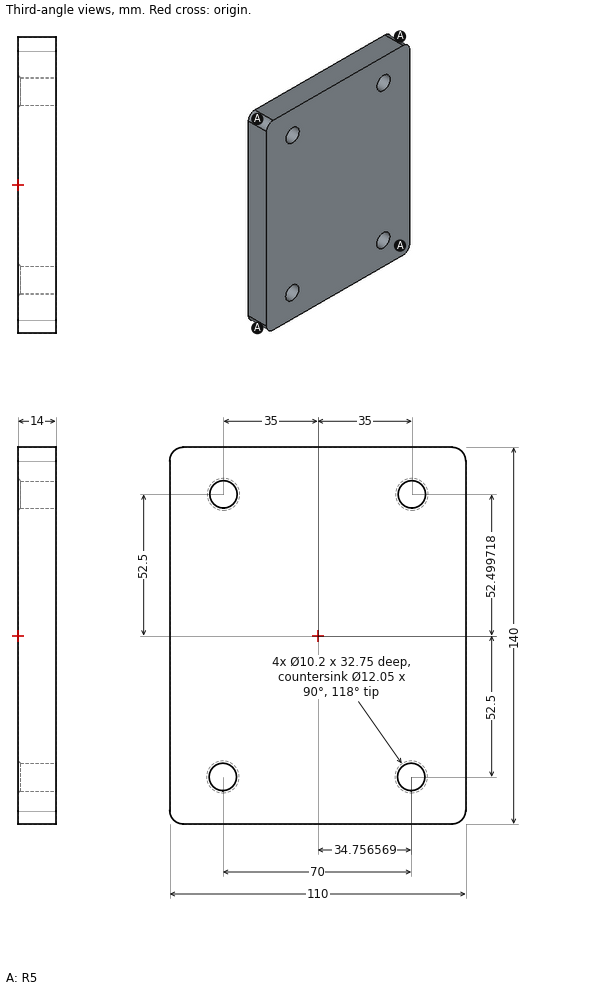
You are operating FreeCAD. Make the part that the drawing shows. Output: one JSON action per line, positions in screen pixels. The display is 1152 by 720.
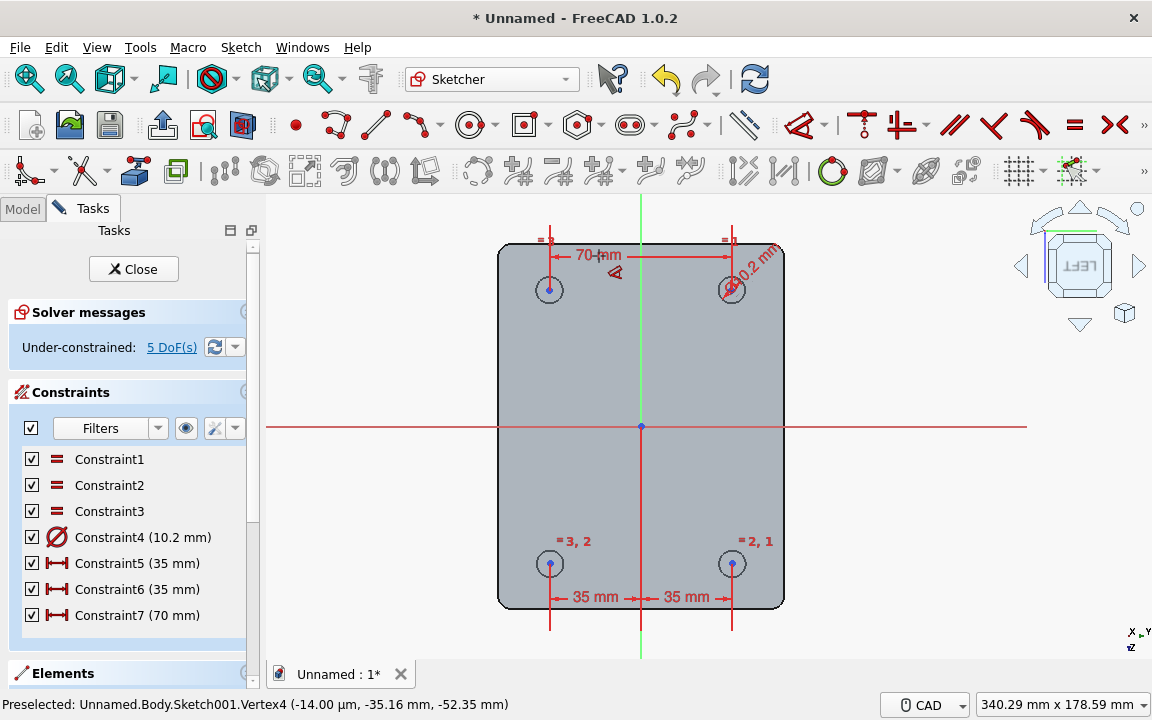
{"action": "left_click", "coordinate": [732, 290]}
{"action": "left_click", "coordinate": [766, 358]}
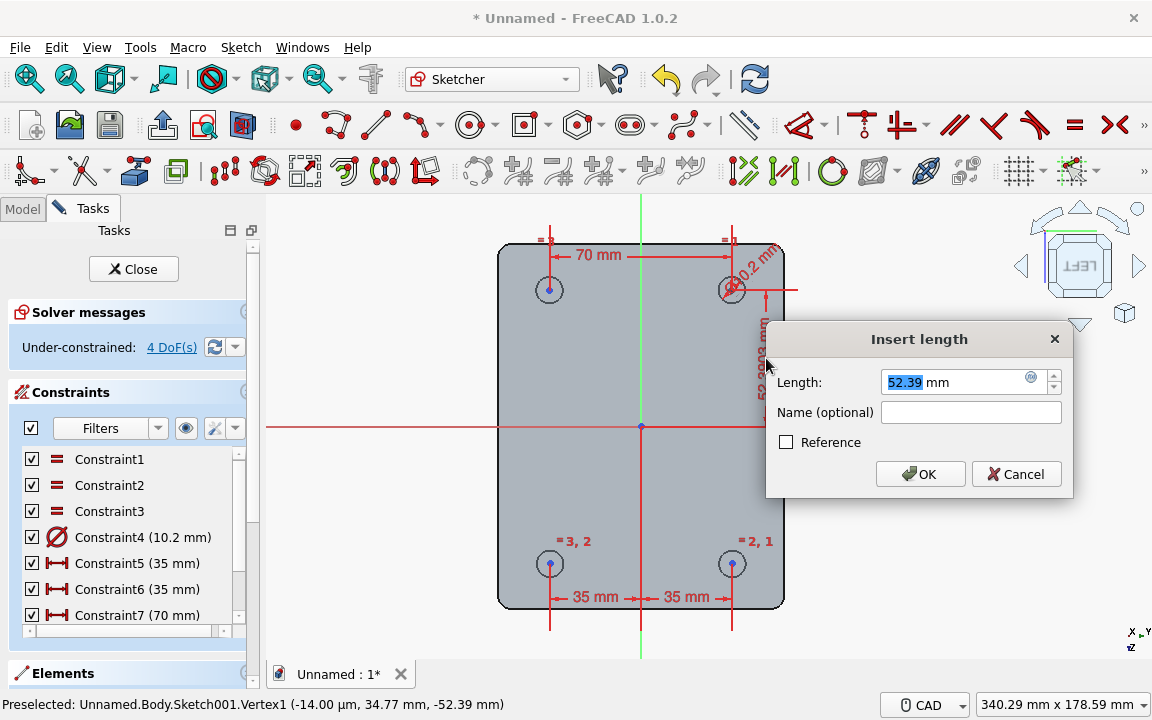
{"action": "type", "text": "52.5"}
{"action": "key", "text": "Return"}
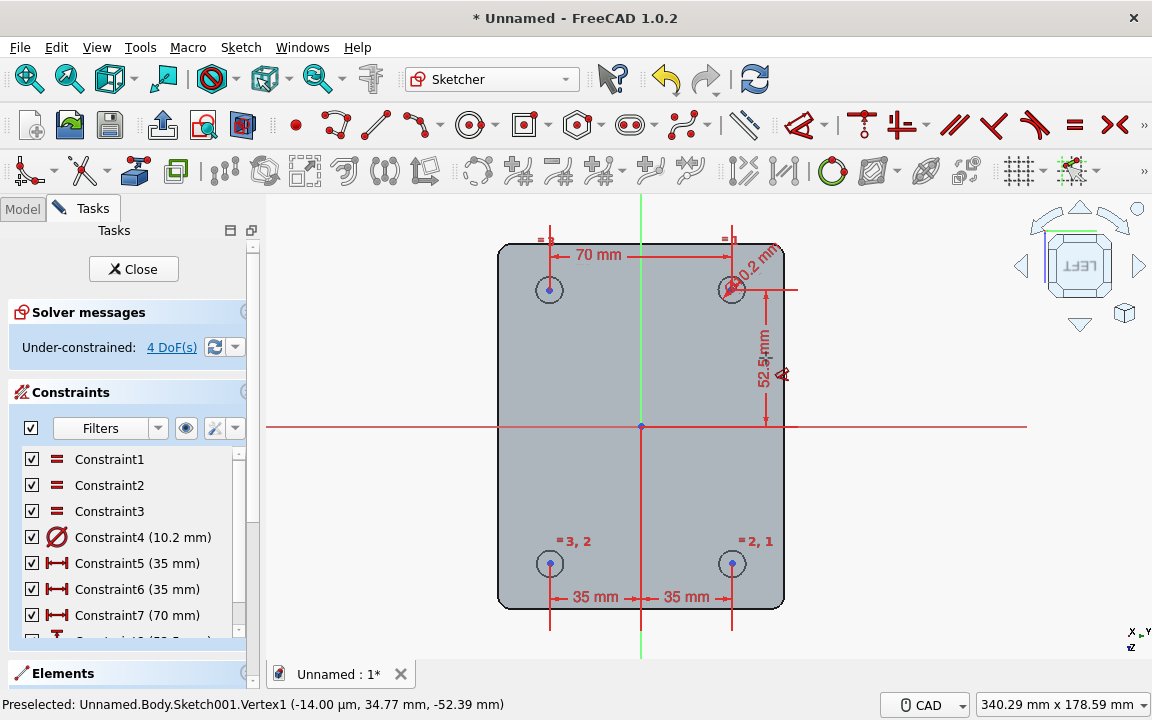
{"action": "left_click", "coordinate": [550, 564]}
{"action": "left_click", "coordinate": [516, 495]}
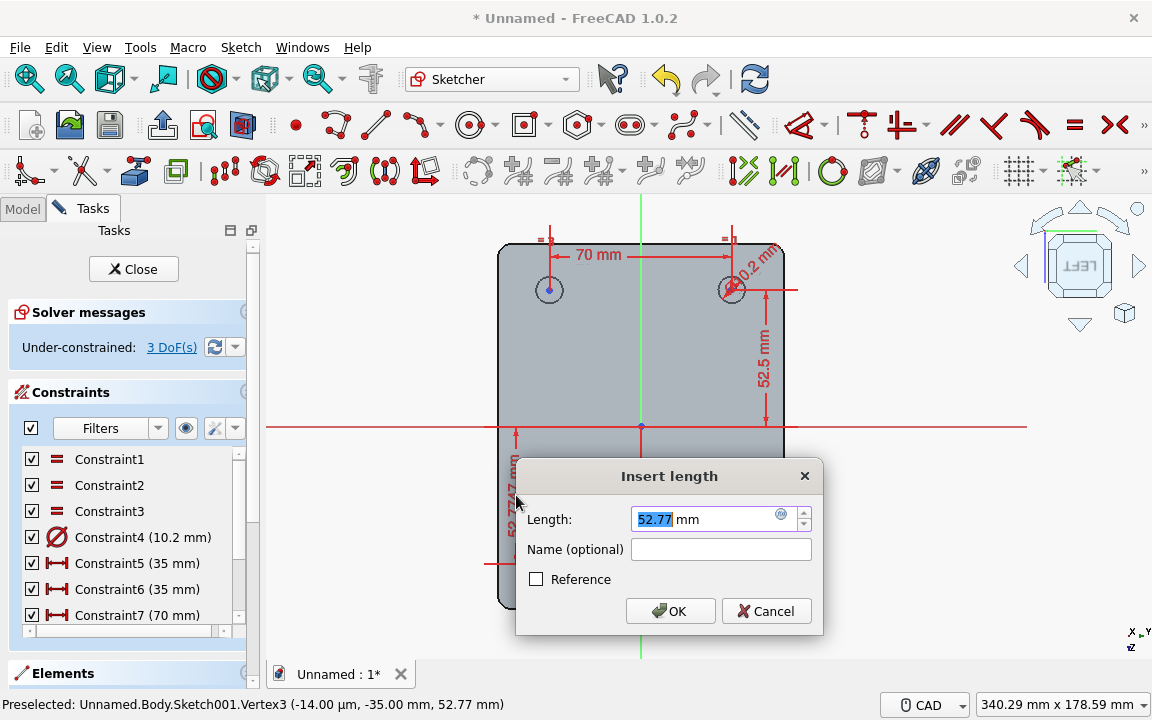
{"action": "type", "text": "52.5"}
{"action": "key", "text": "Return"}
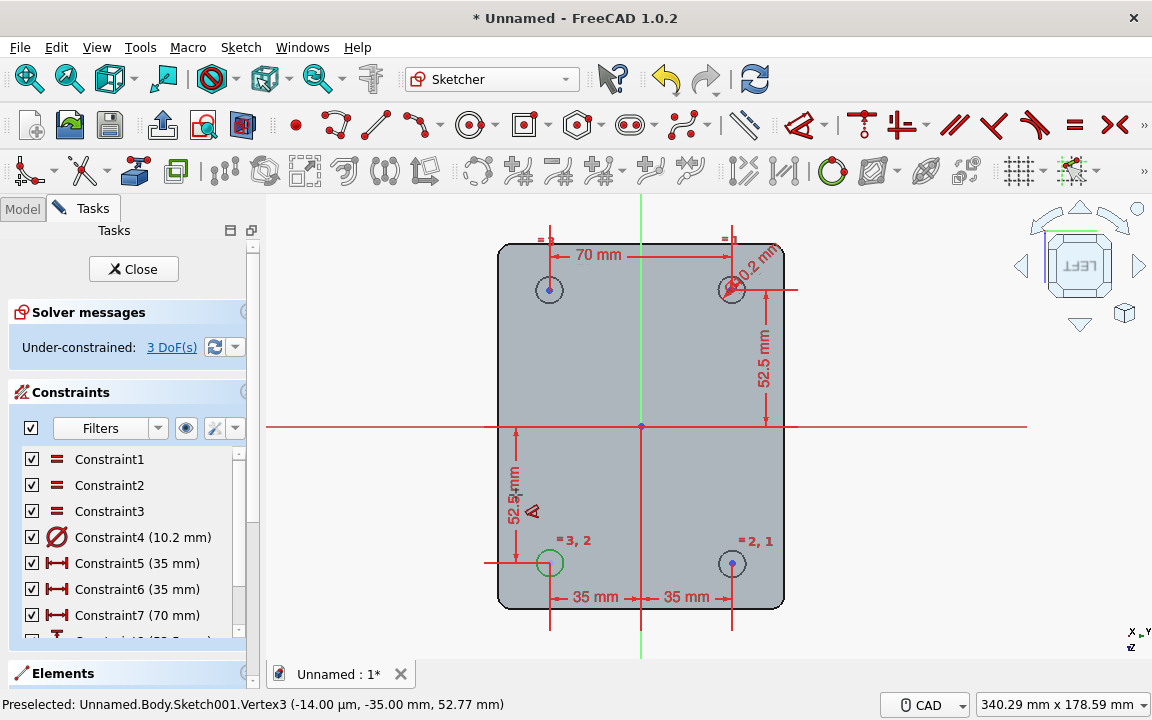
{"action": "left_click", "coordinate": [550, 290]}
{"action": "left_click", "coordinate": [516, 358]}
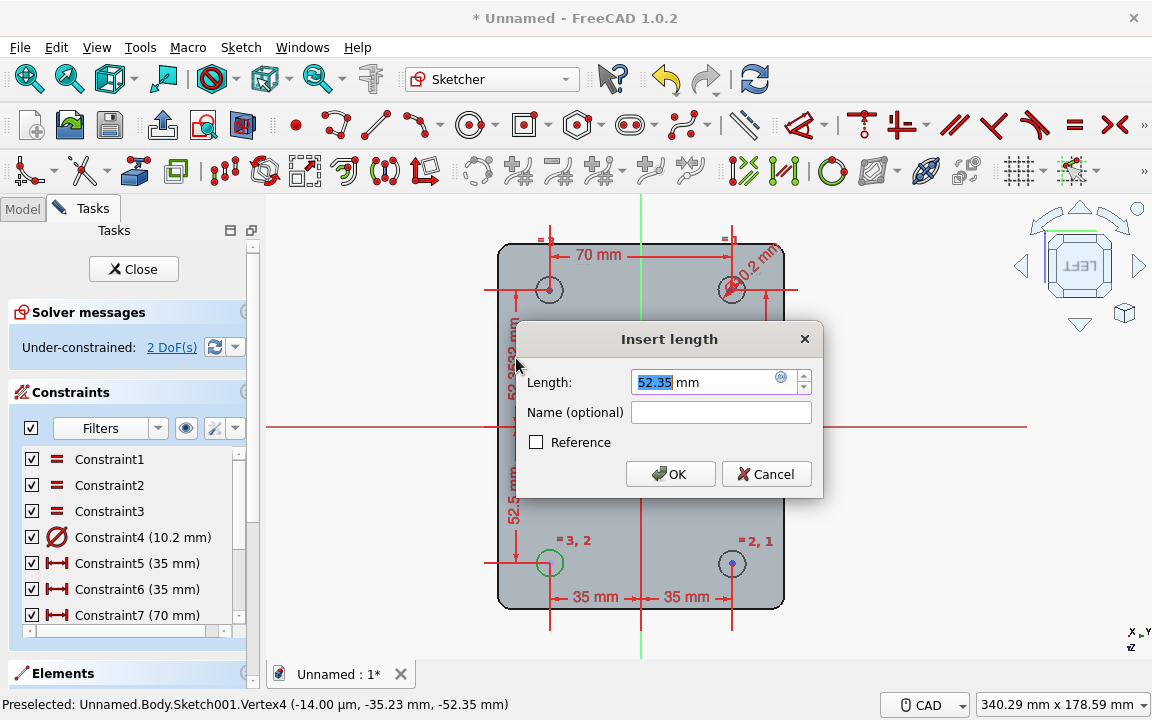
{"action": "type", "text": "52.5"}
{"action": "key", "text": "Return"}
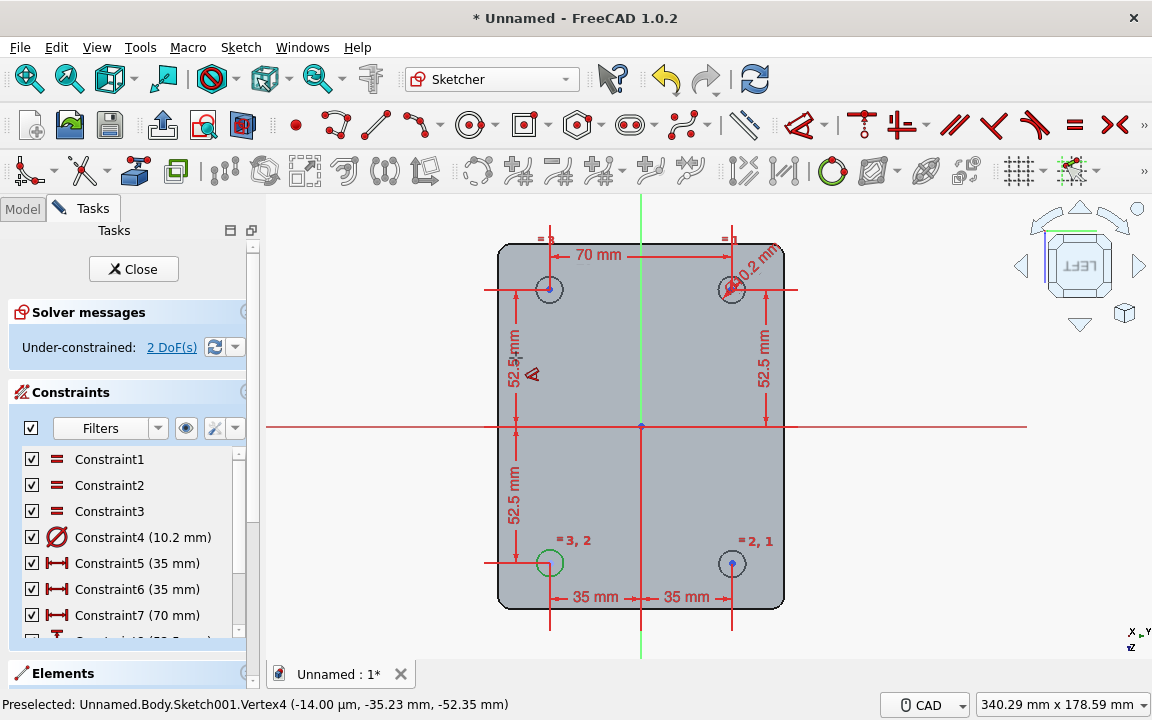
{"action": "left_click", "coordinate": [732, 290]}
{"action": "left_click", "coordinate": [687, 460]}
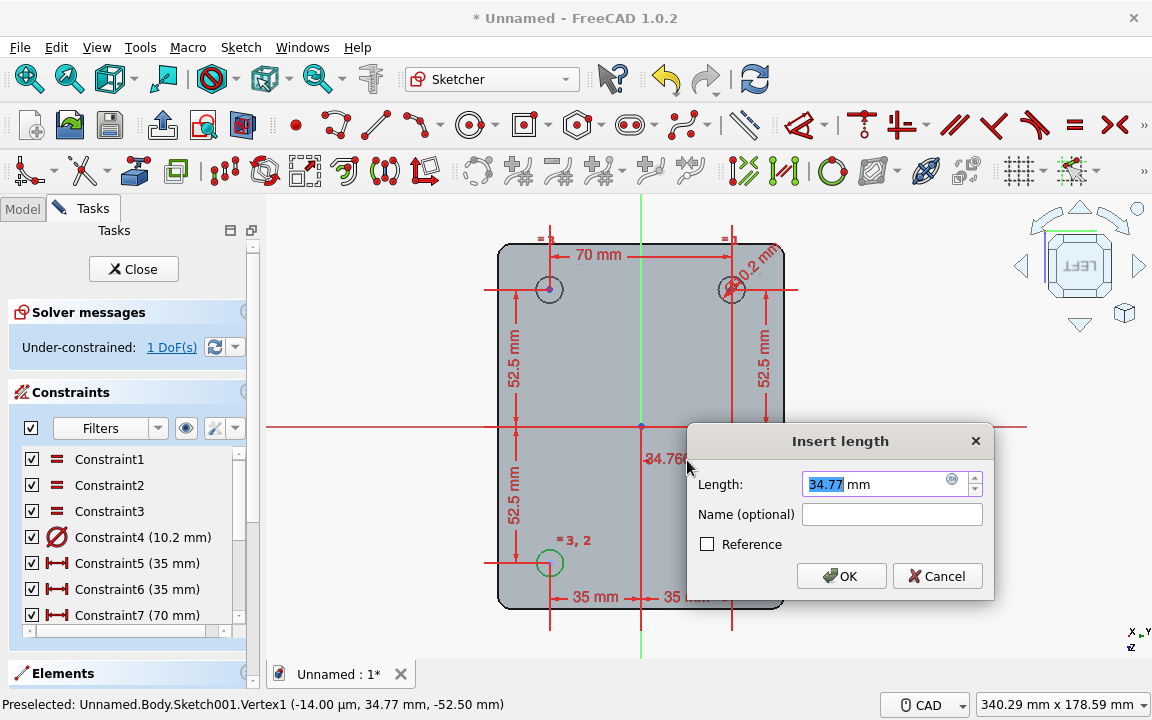
{"action": "type", "text": "34.756569"}
{"action": "key", "text": "Return"}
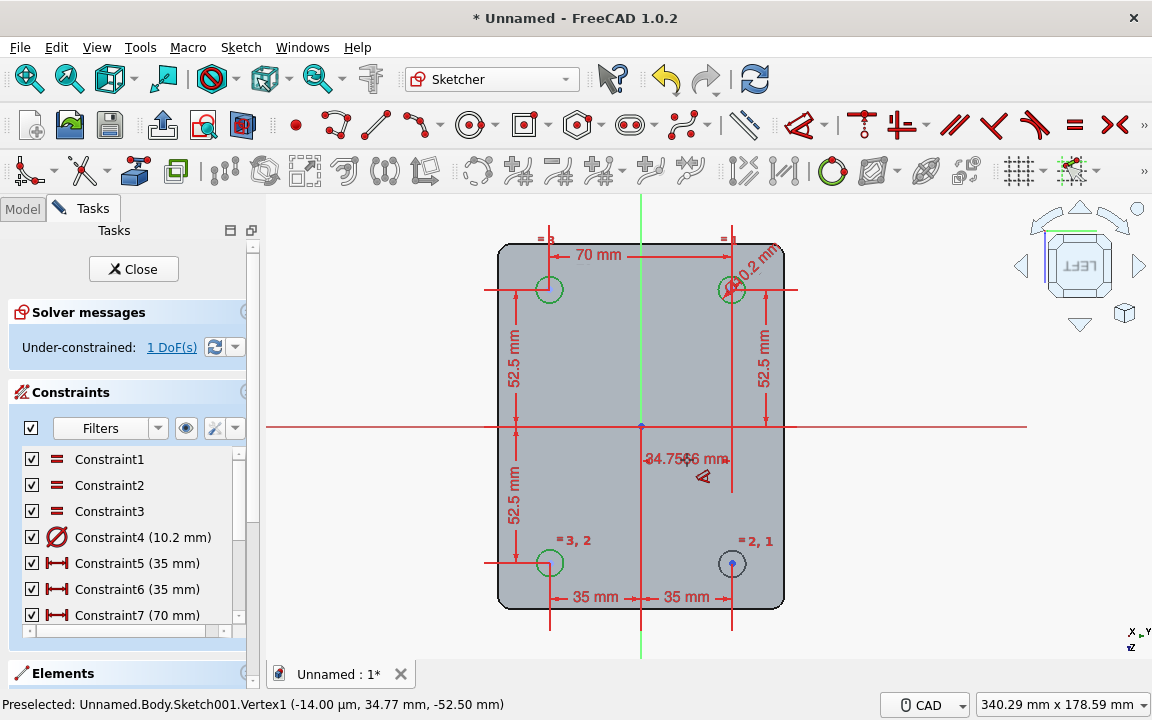
{"action": "left_click", "coordinate": [732, 564]}
{"action": "left_click", "coordinate": [766, 495]}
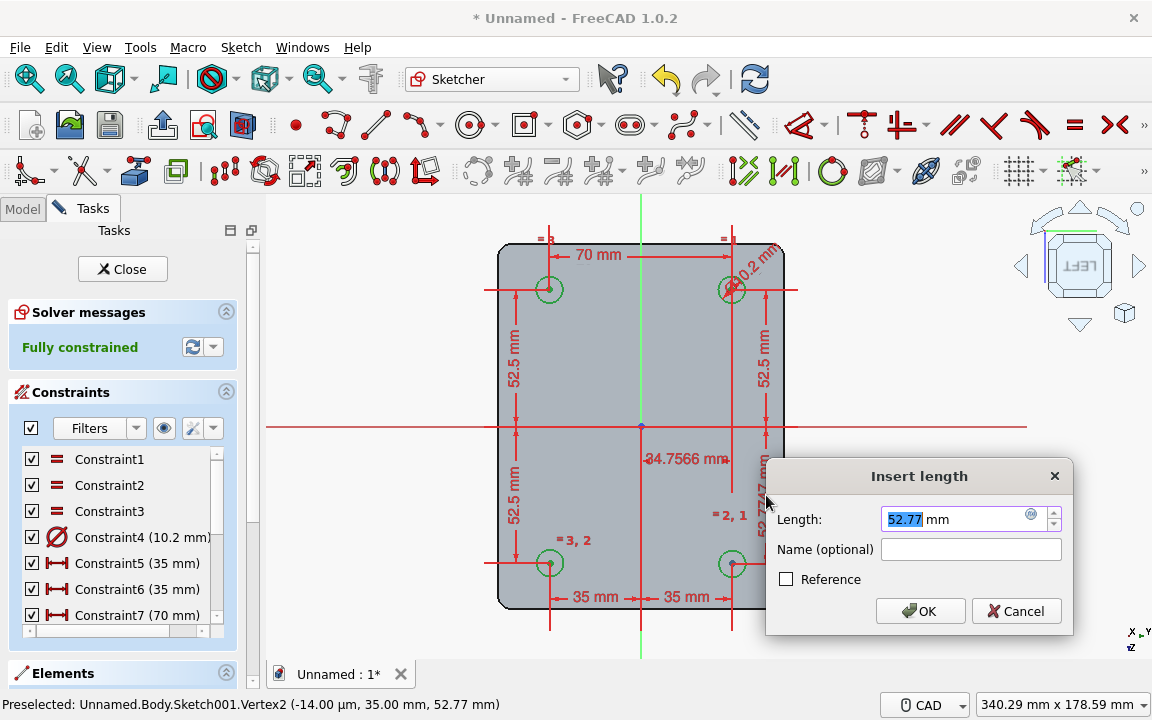
{"action": "type", "text": "52.499718"}
{"action": "key", "text": "Return"}
{"action": "key", "text": "Escape"}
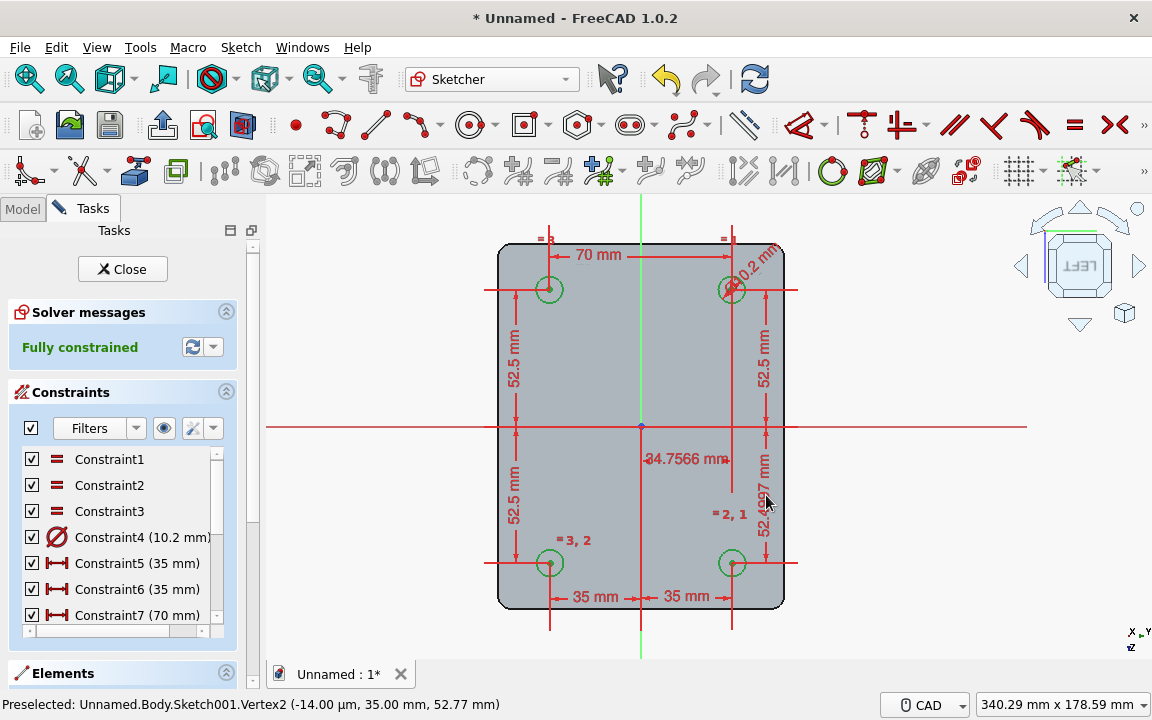
{"action": "left_click", "coordinate": [123, 269]}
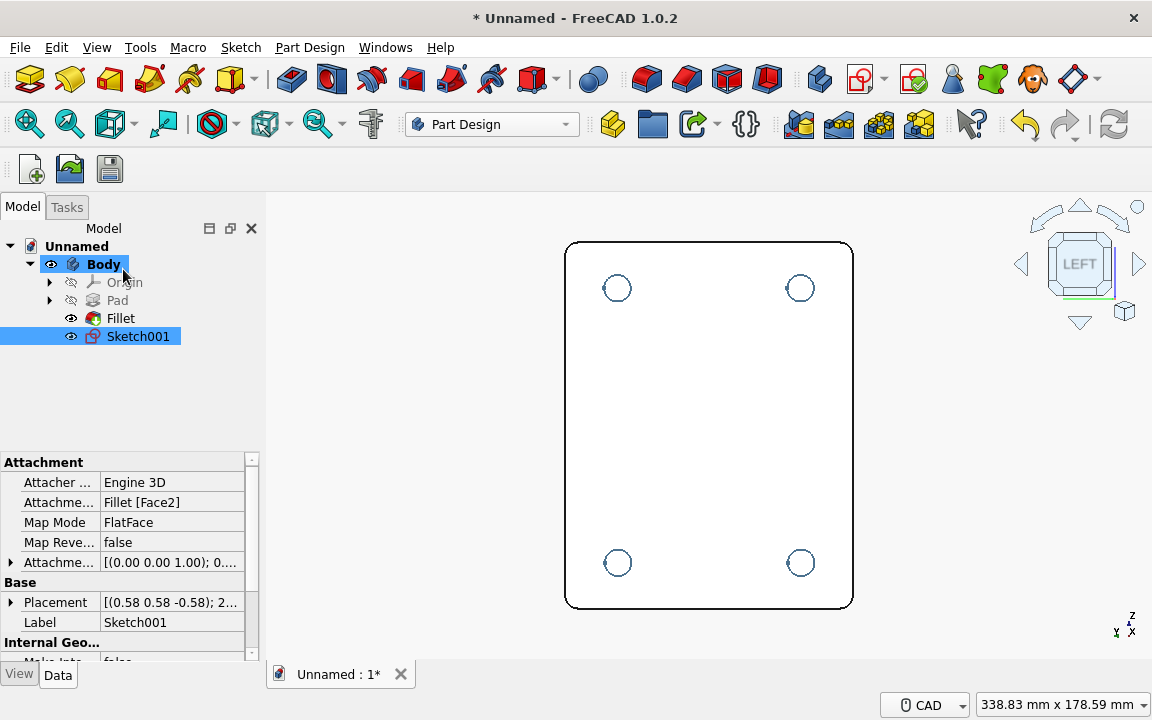
{"action": "left_click", "coordinate": [332, 80]}